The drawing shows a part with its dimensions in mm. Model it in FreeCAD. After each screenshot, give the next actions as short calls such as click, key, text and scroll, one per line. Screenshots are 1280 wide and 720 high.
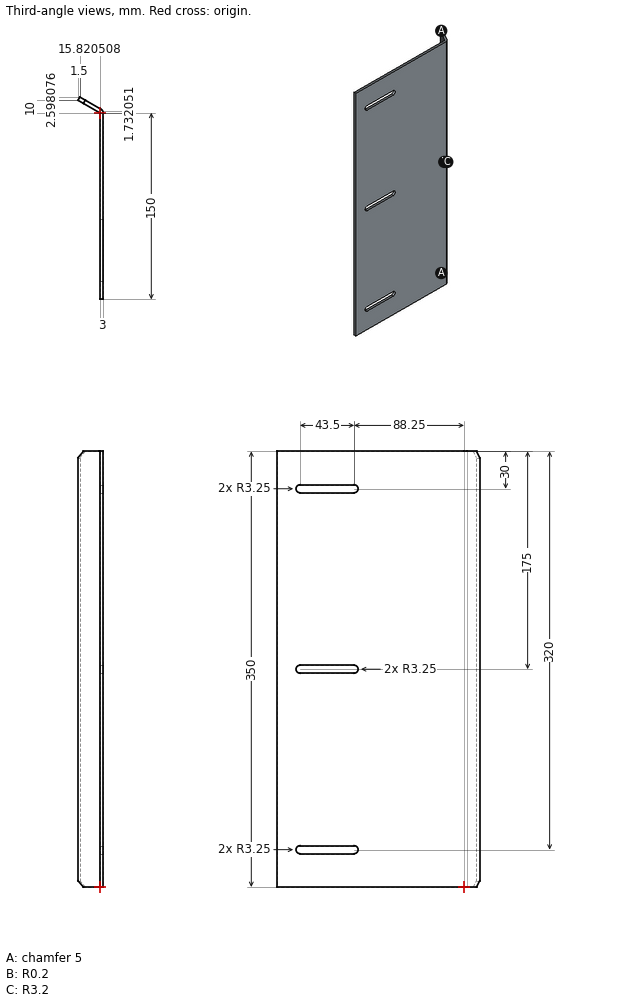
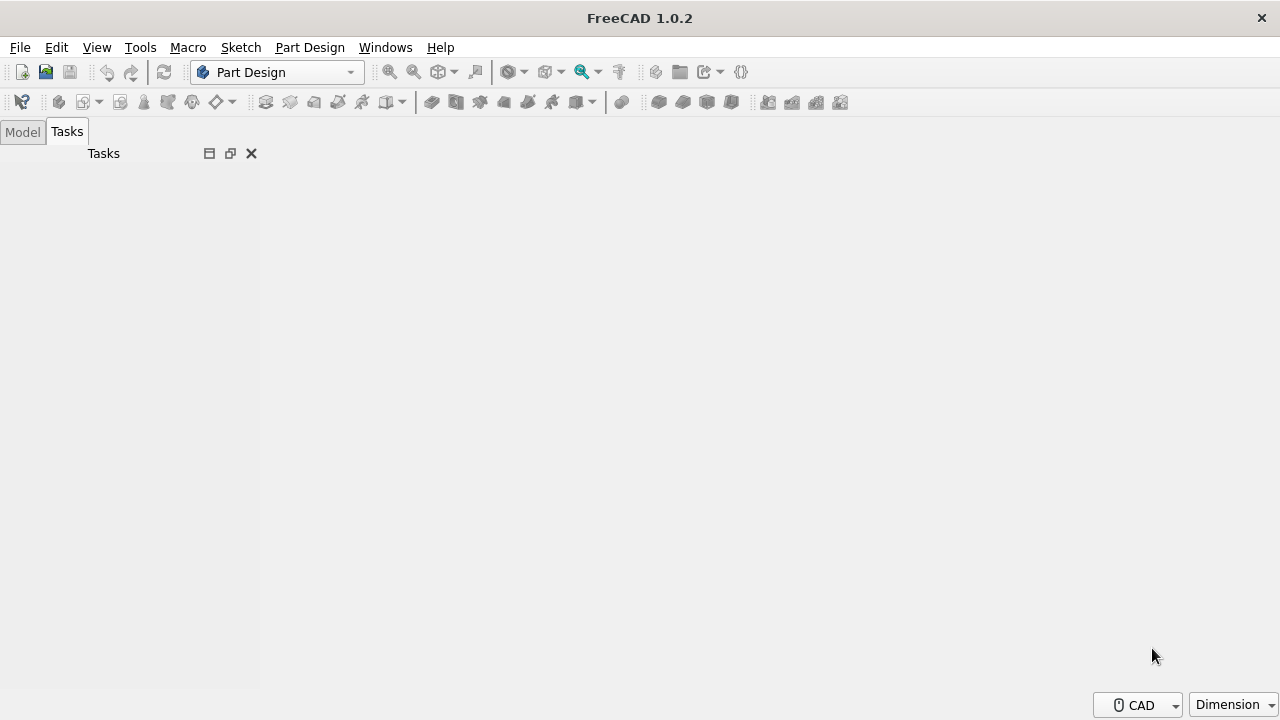
click(22, 72)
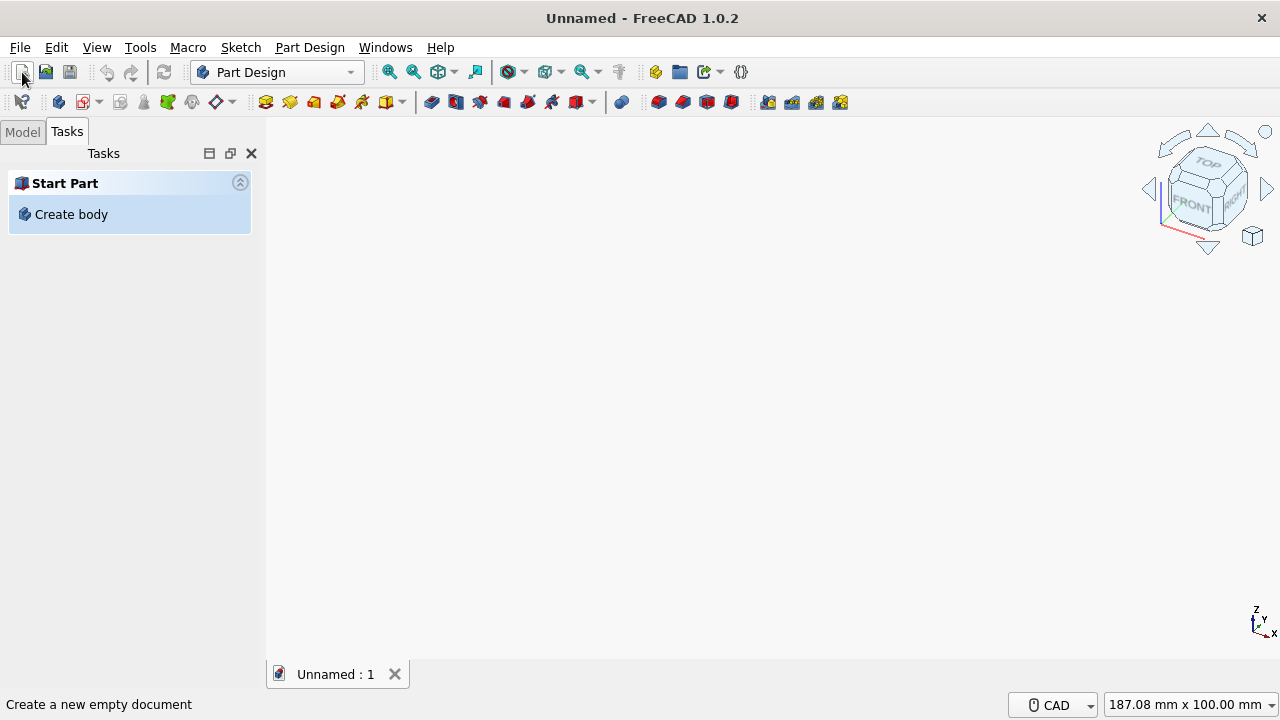
click(60, 102)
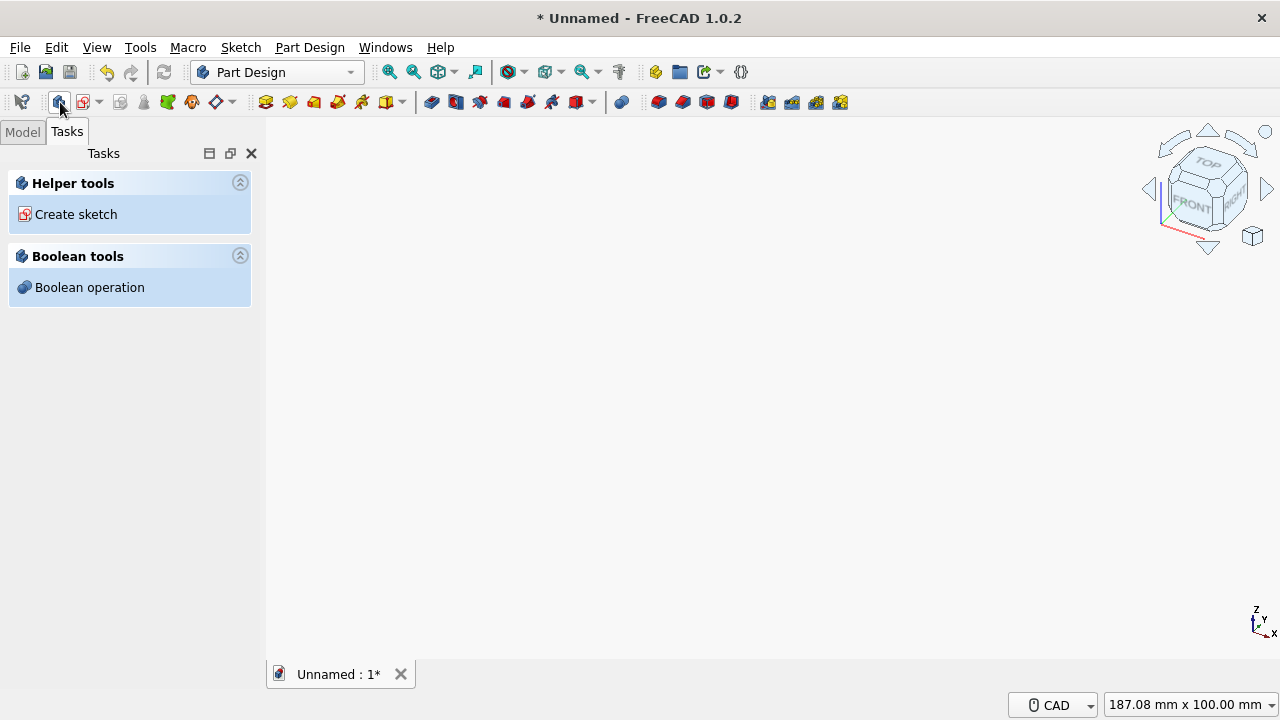
click(23, 131)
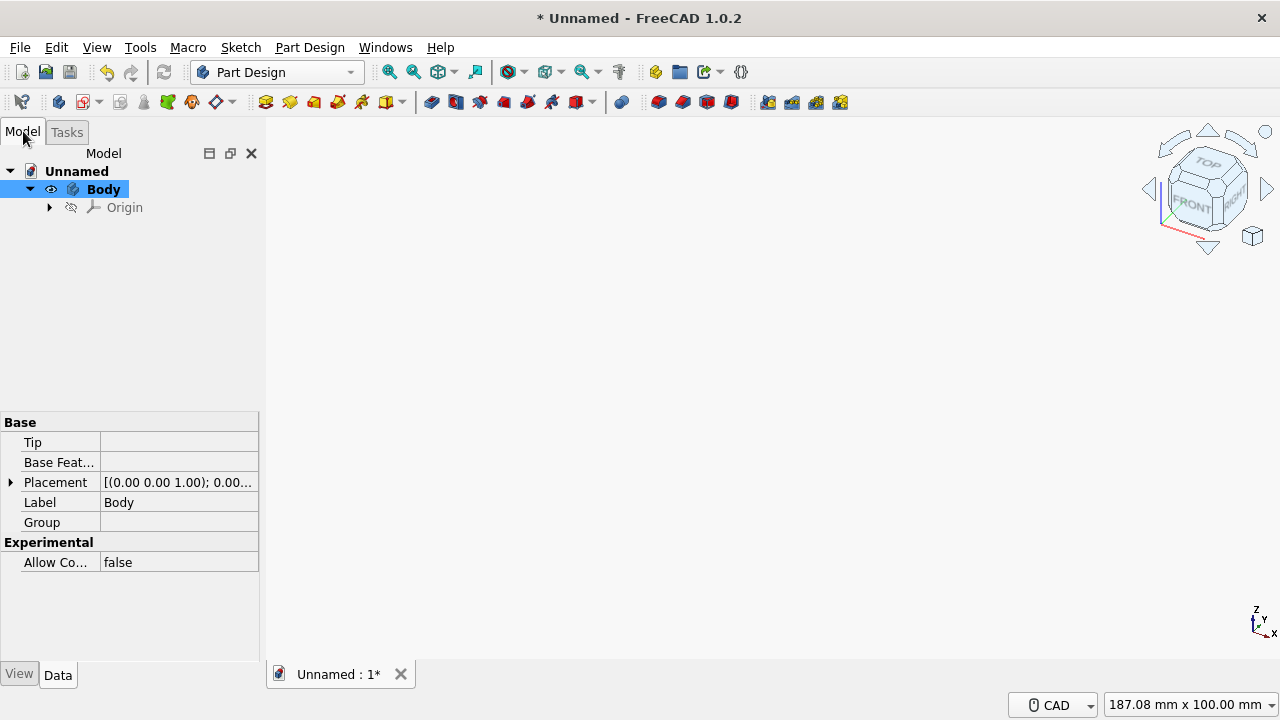
click(50, 207)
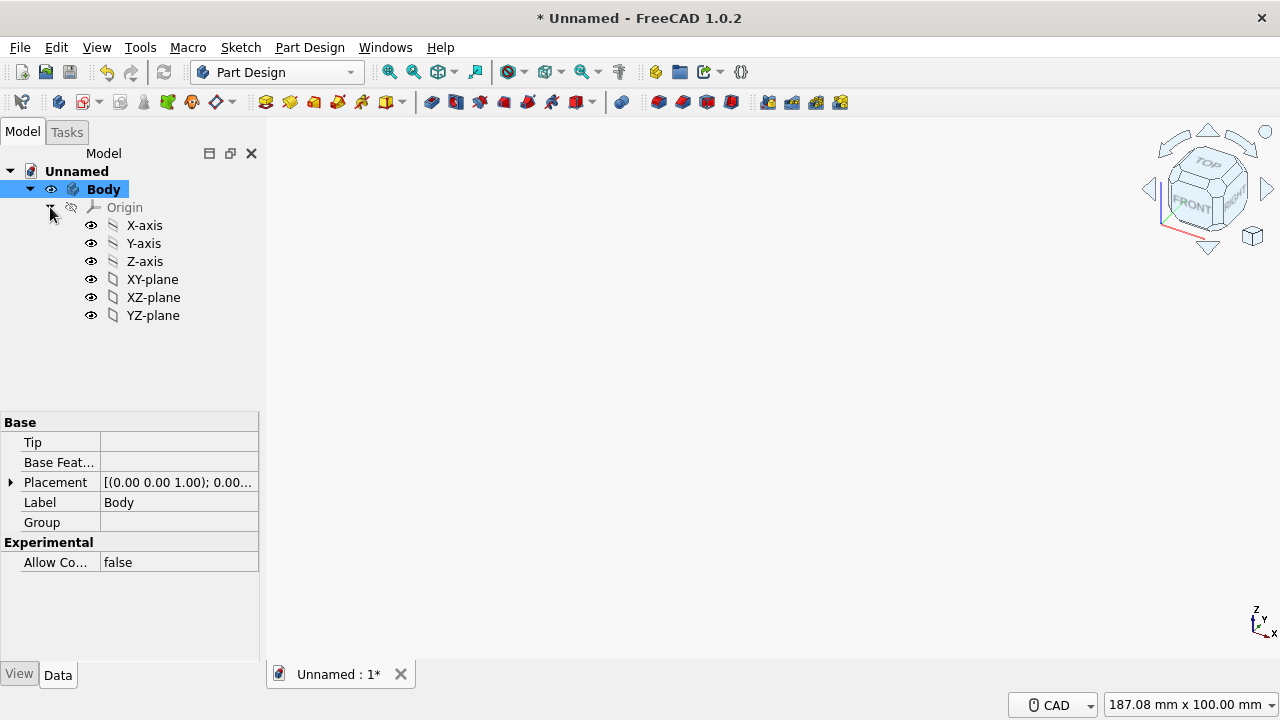
click(136, 279)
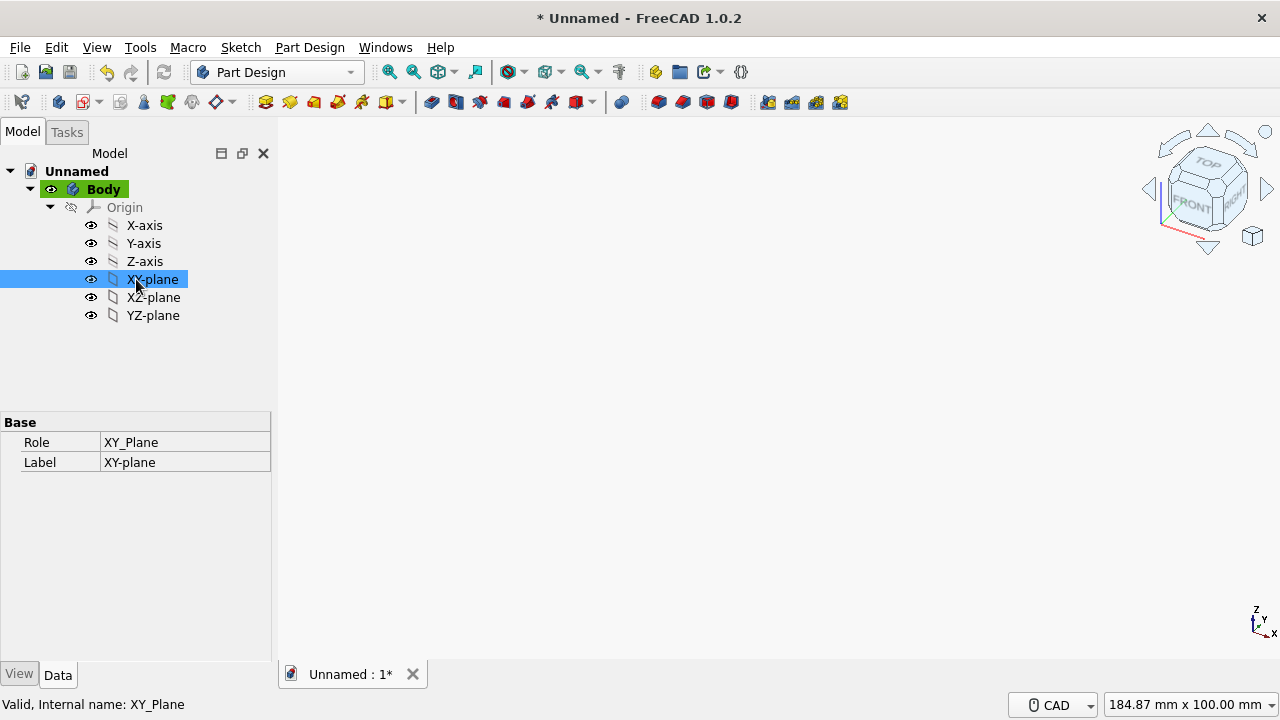
click(216, 102)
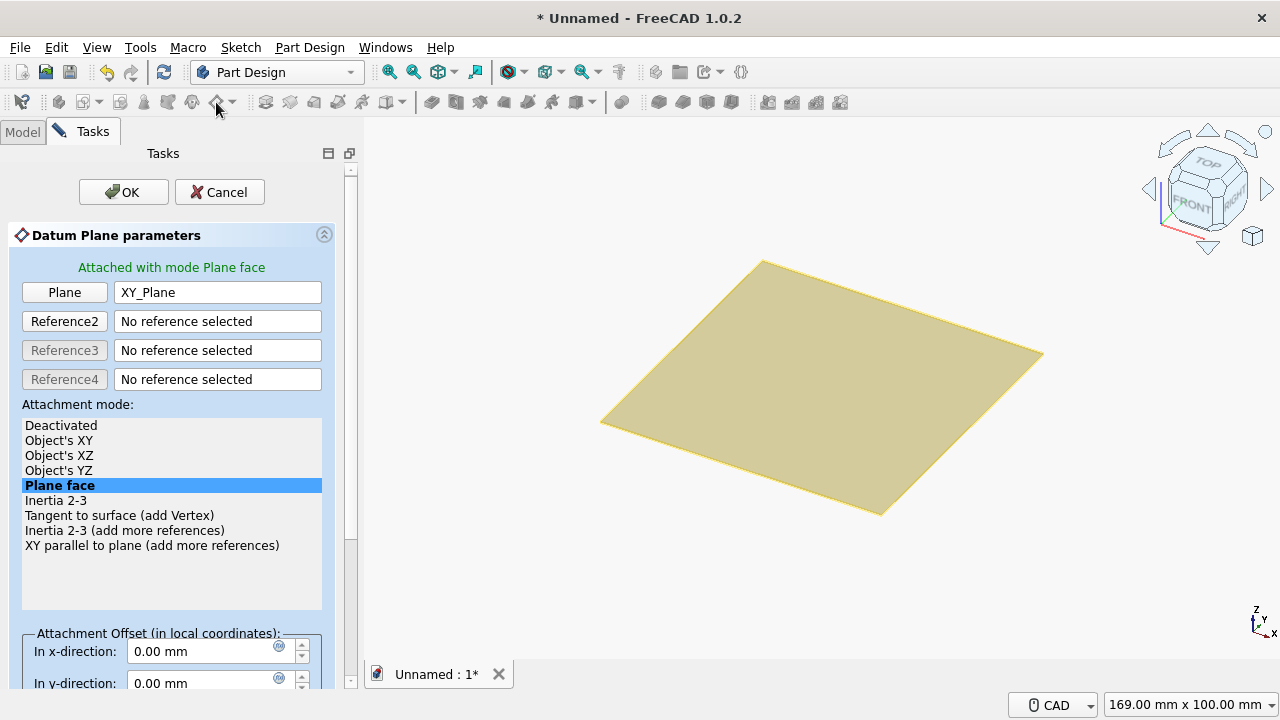
scroll(351, 426, down, 2)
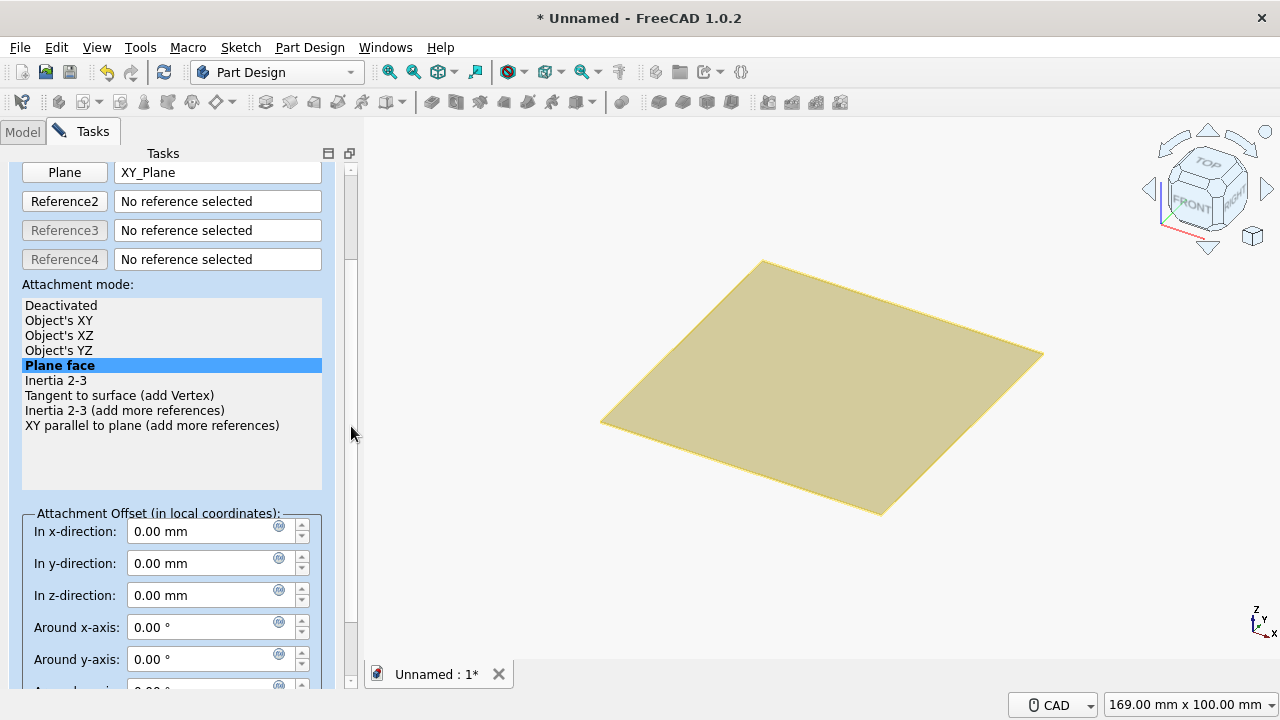
triple_click(210, 595)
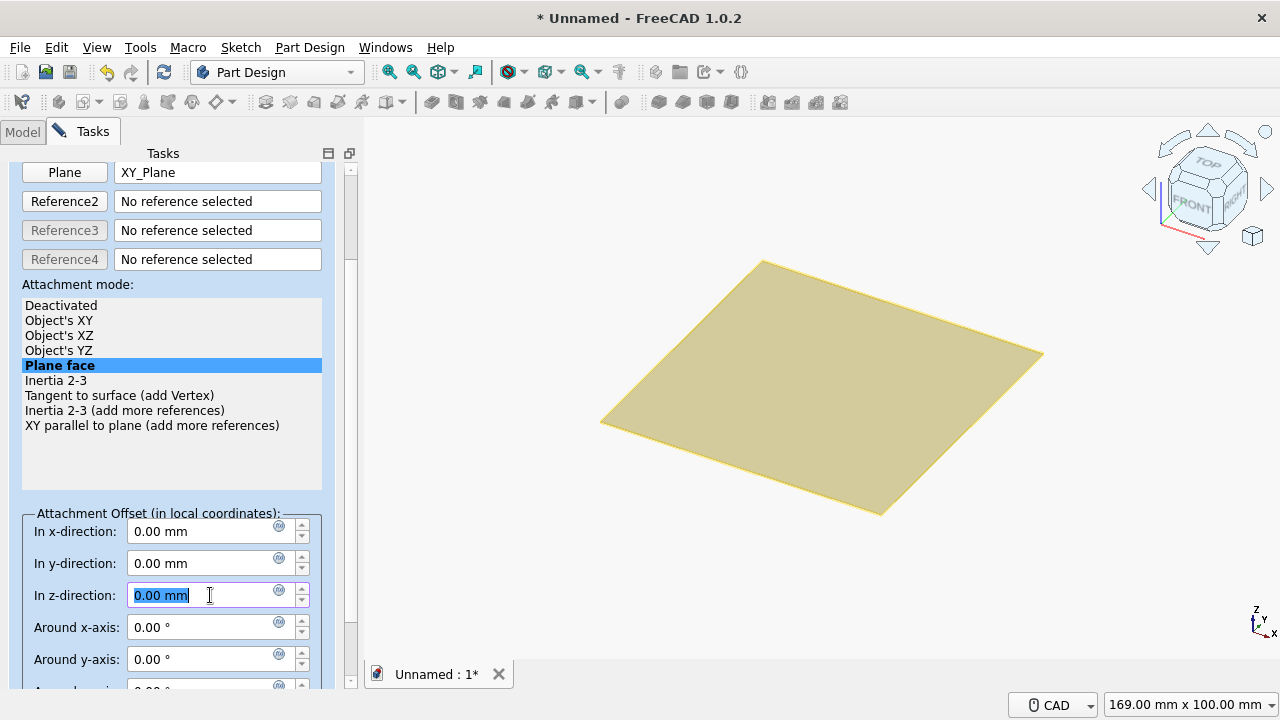
text(350)
key(Tab)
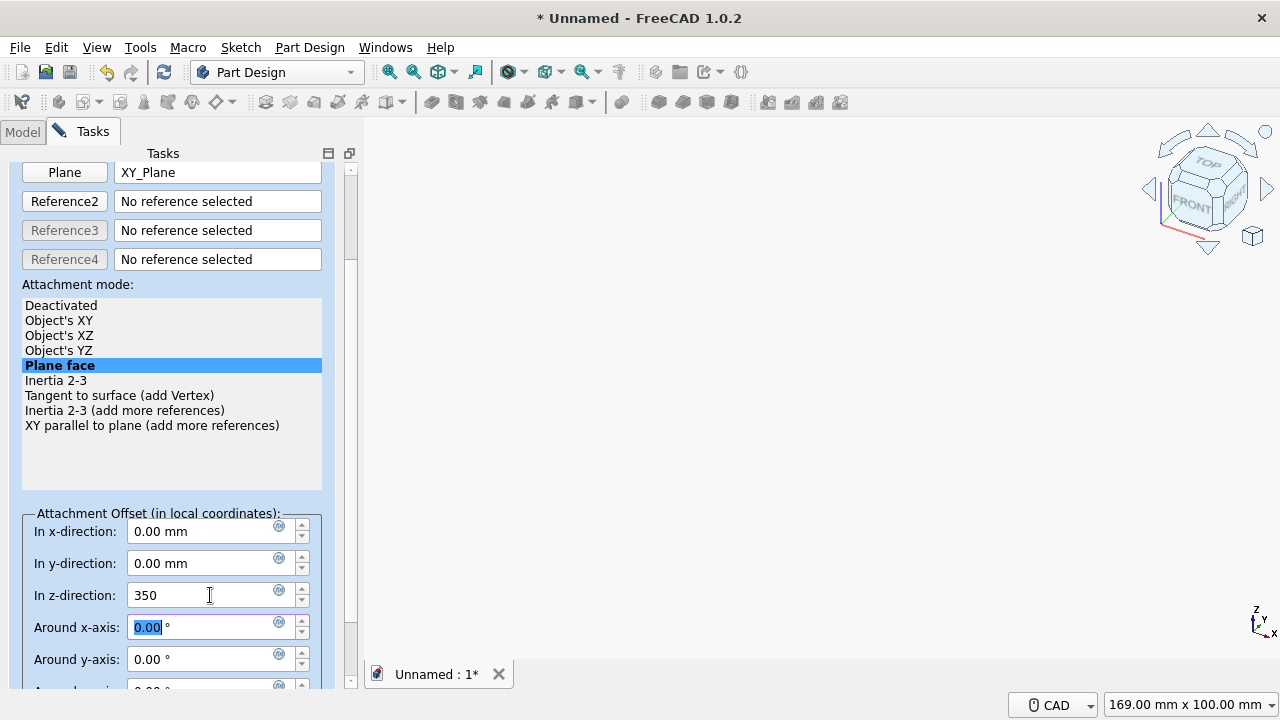
scroll(351, 426, up, 3)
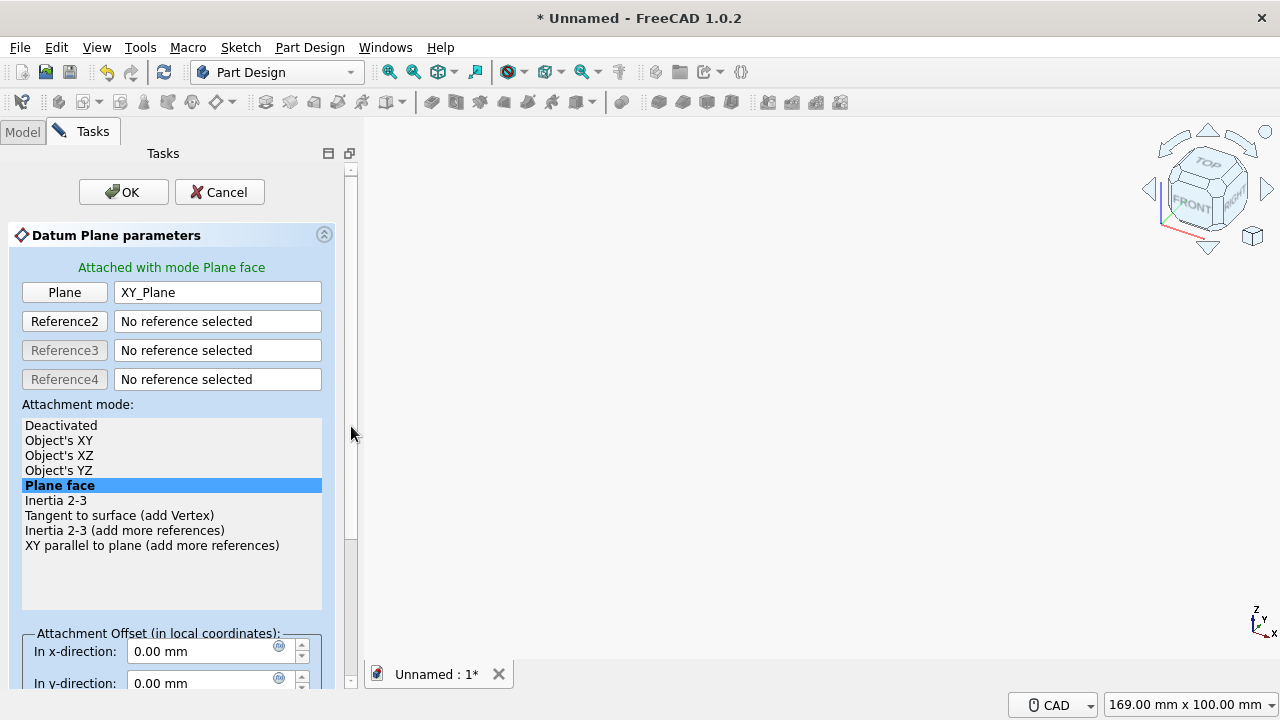
click(124, 192)